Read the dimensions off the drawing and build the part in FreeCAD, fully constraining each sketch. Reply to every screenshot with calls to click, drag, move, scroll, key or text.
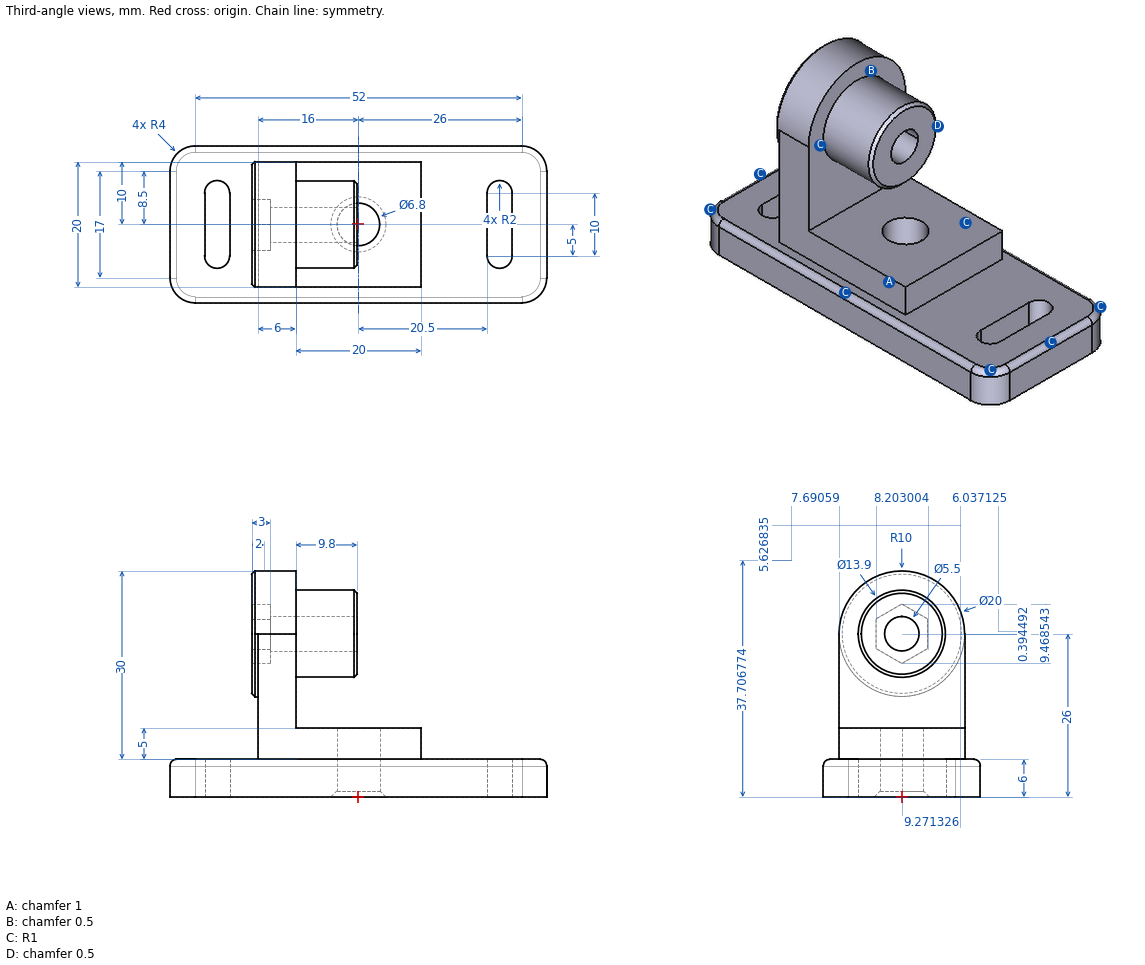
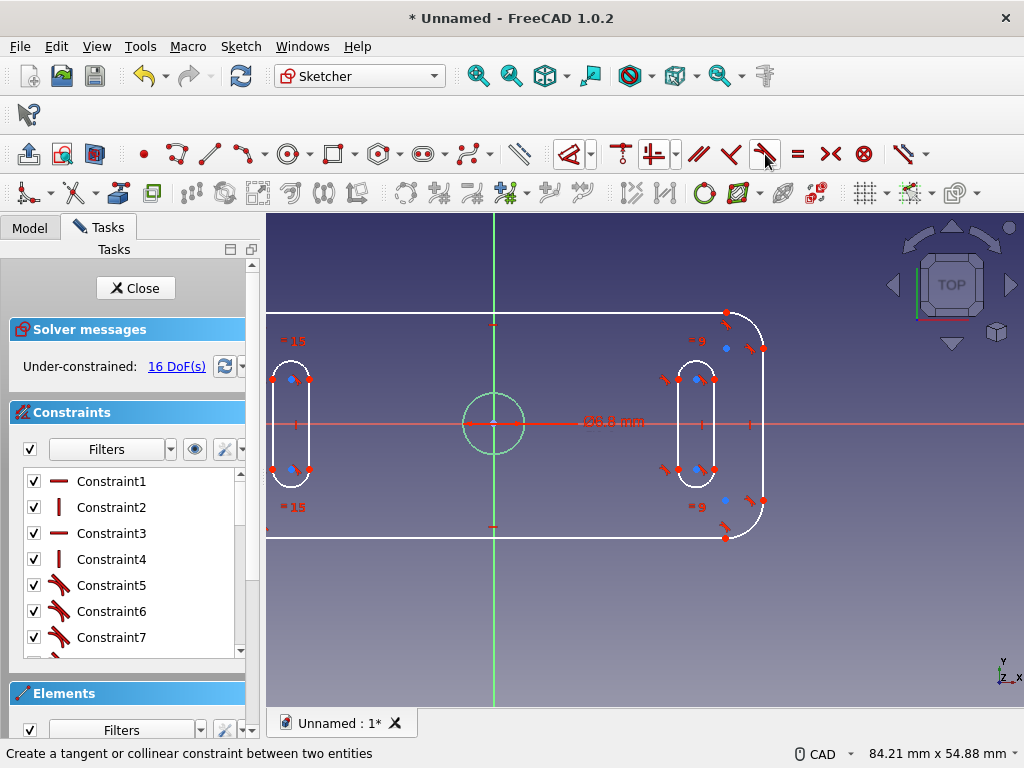
scroll(745, 534, down, 2)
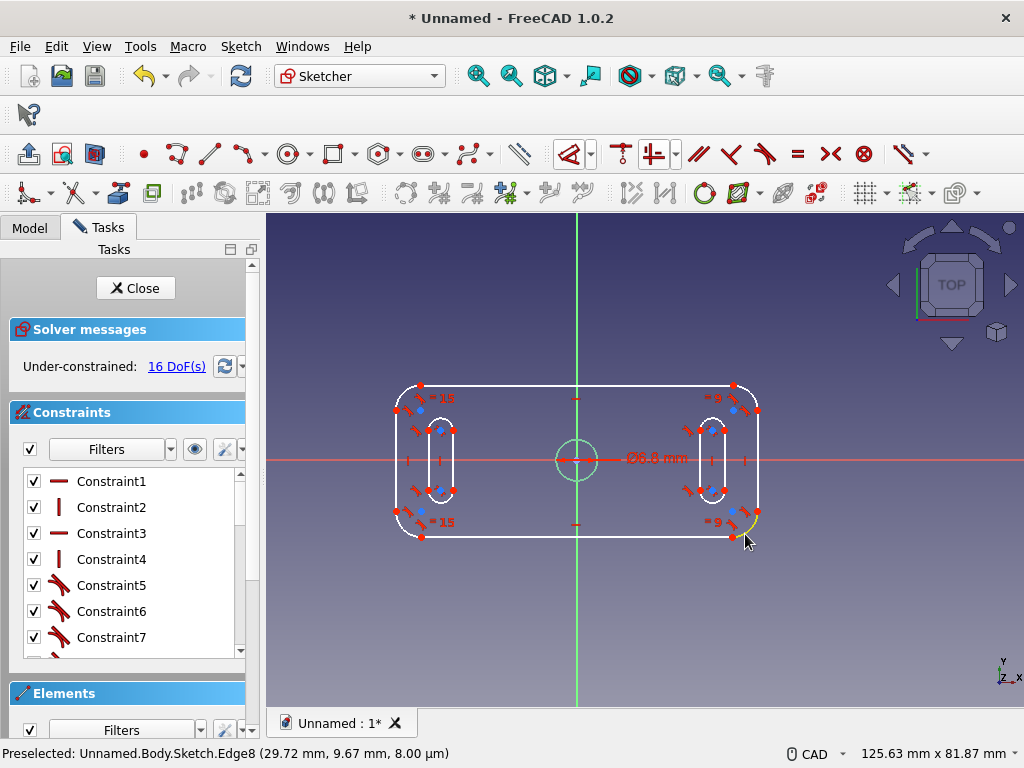
click(409, 388)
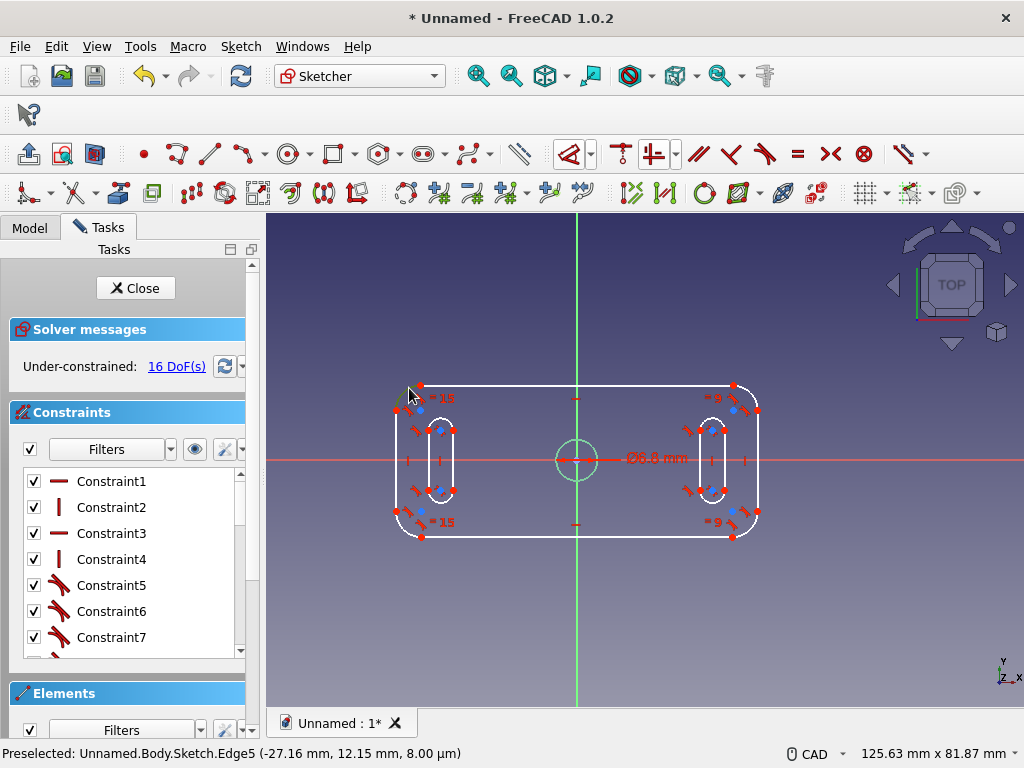
click(399, 523)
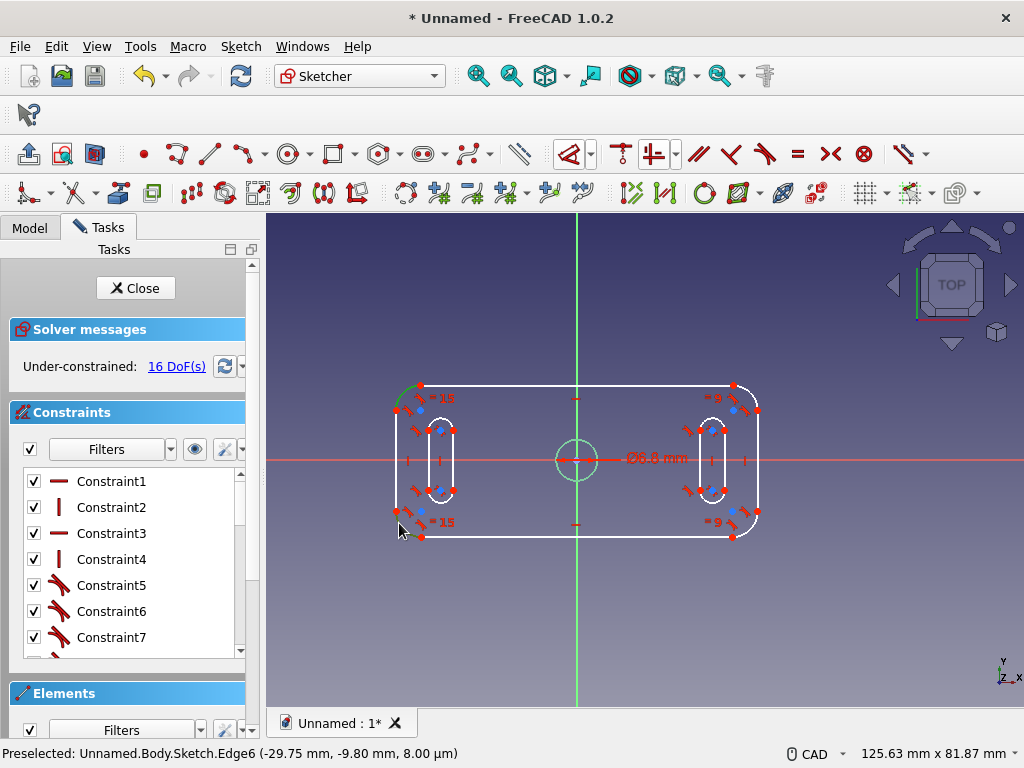
click(744, 534)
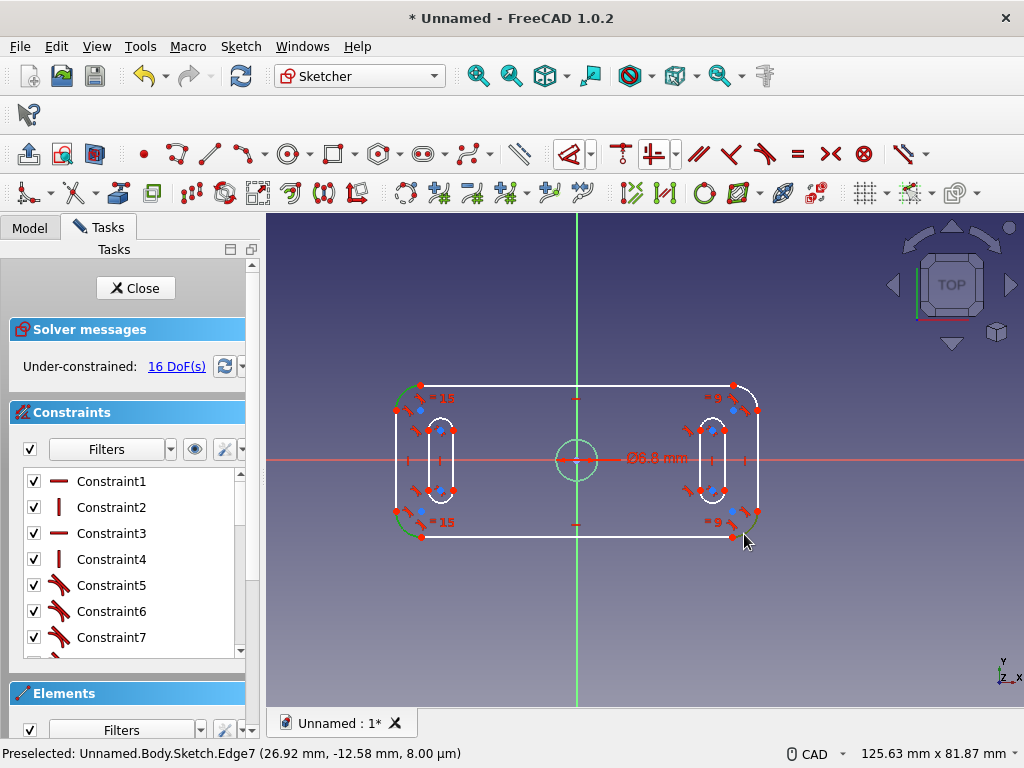
click(755, 399)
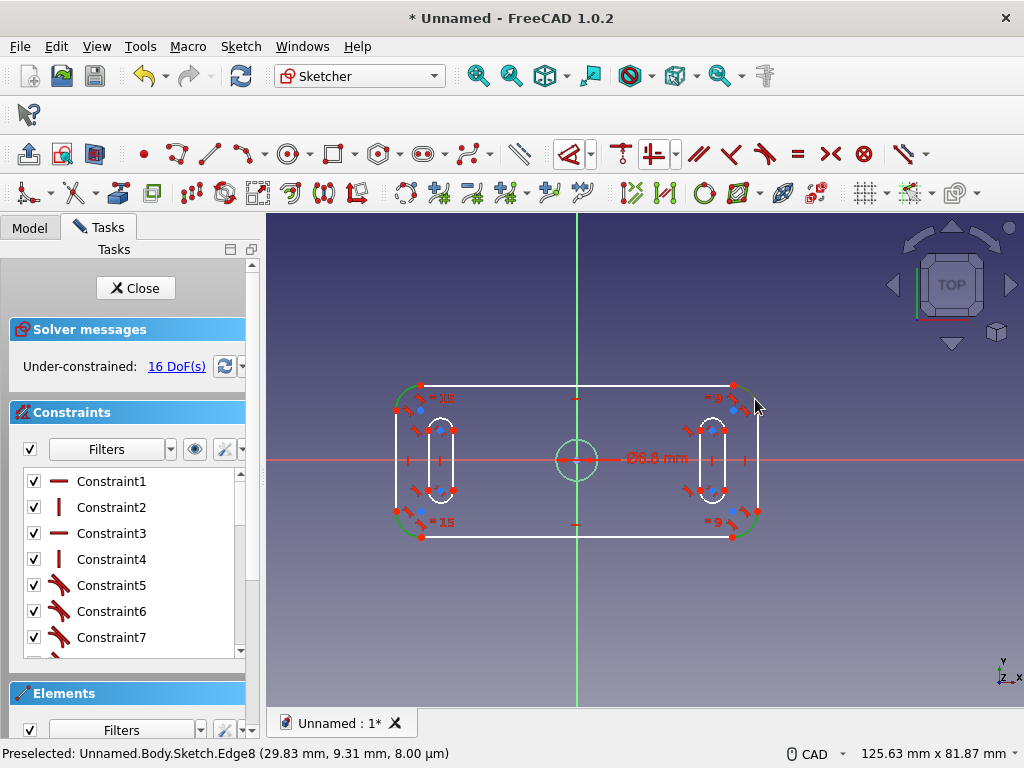
click(798, 154)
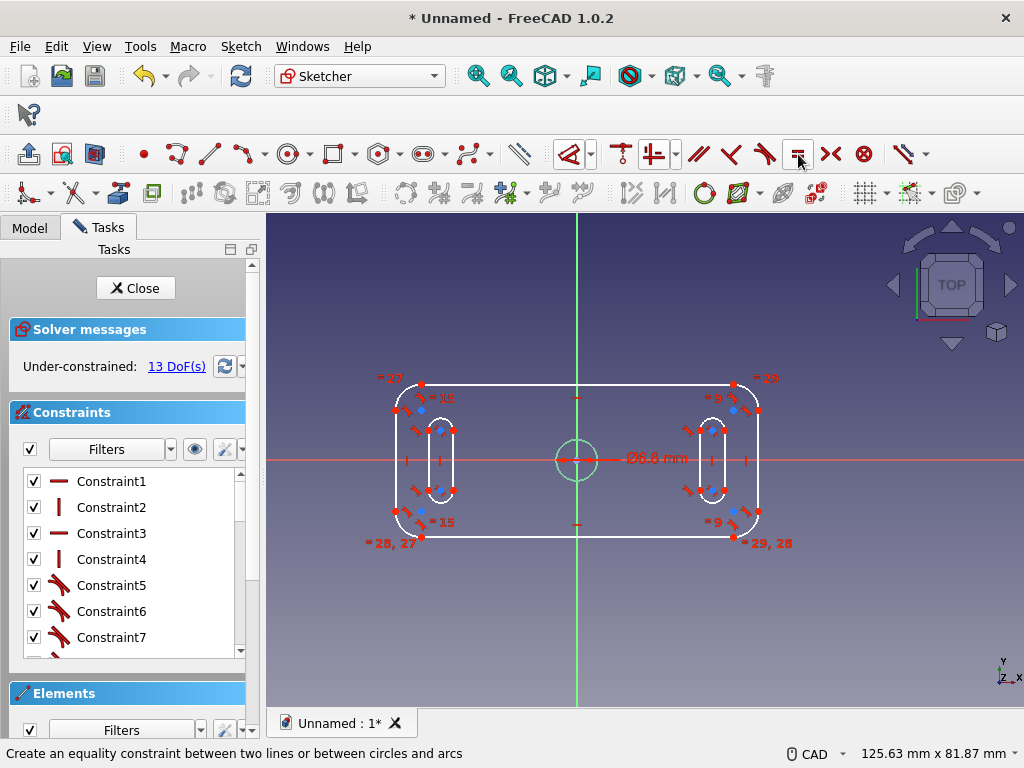
scroll(705, 501, up, 2)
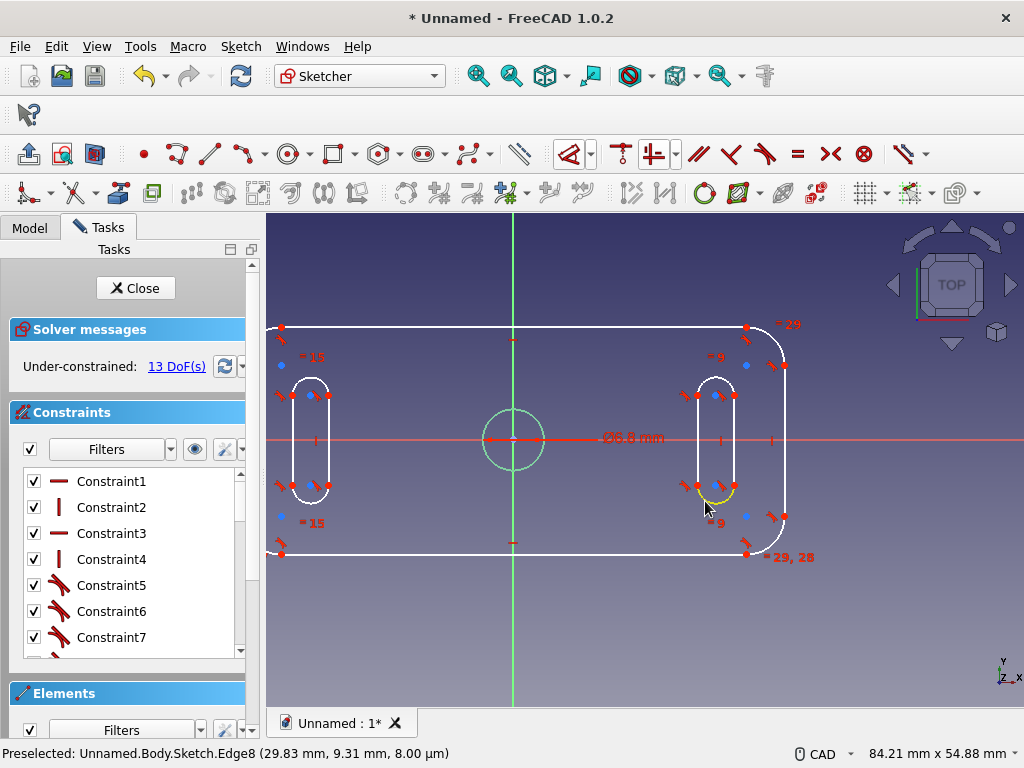
click(705, 500)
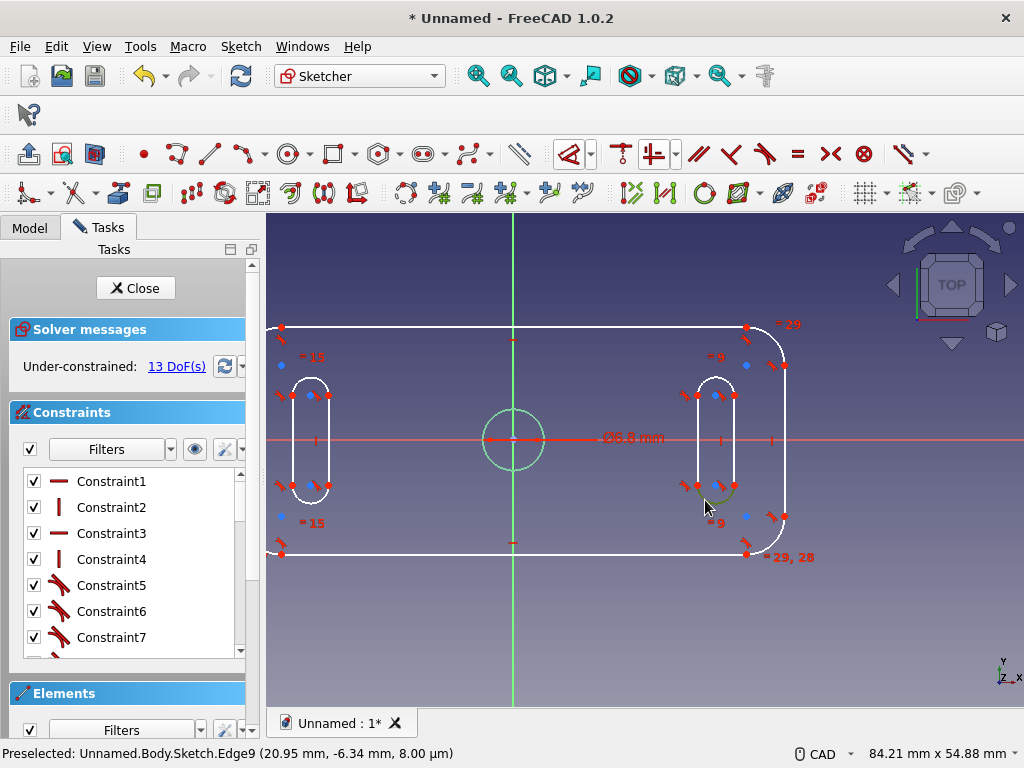
click(300, 500)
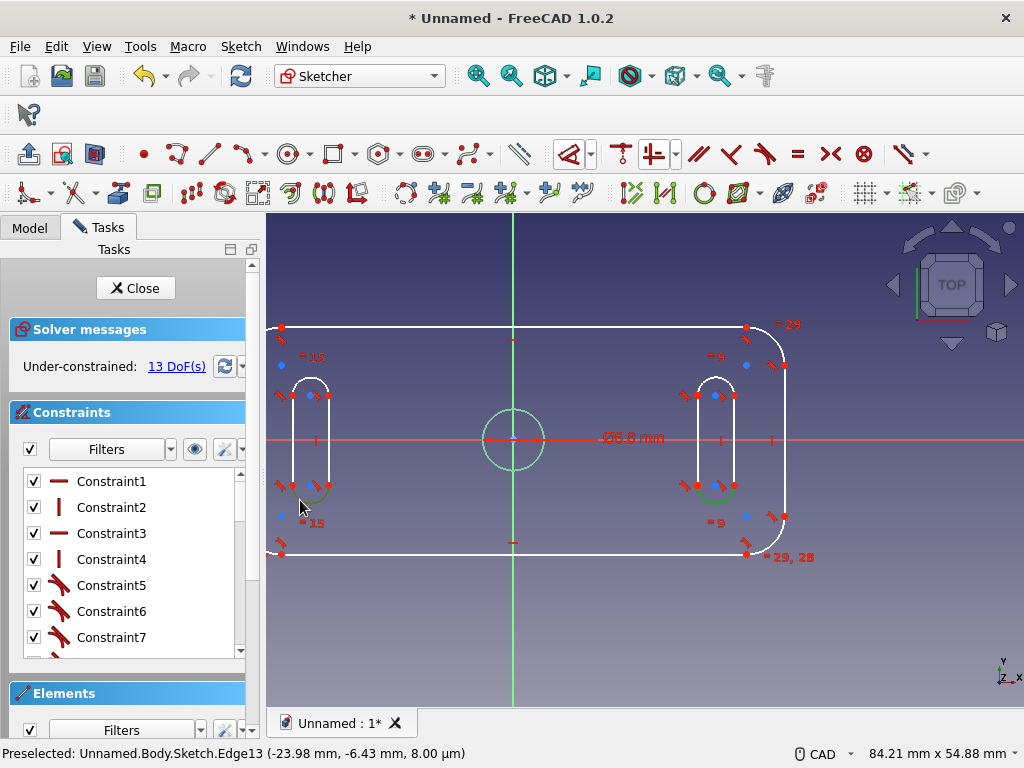
click(798, 154)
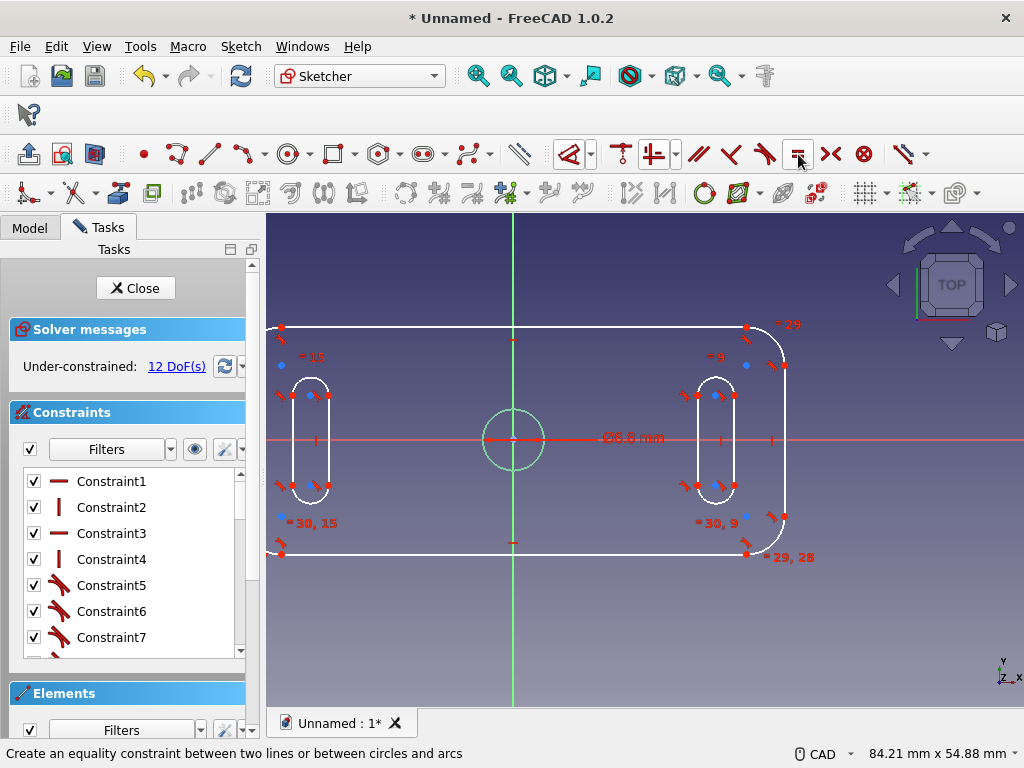
click(716, 486)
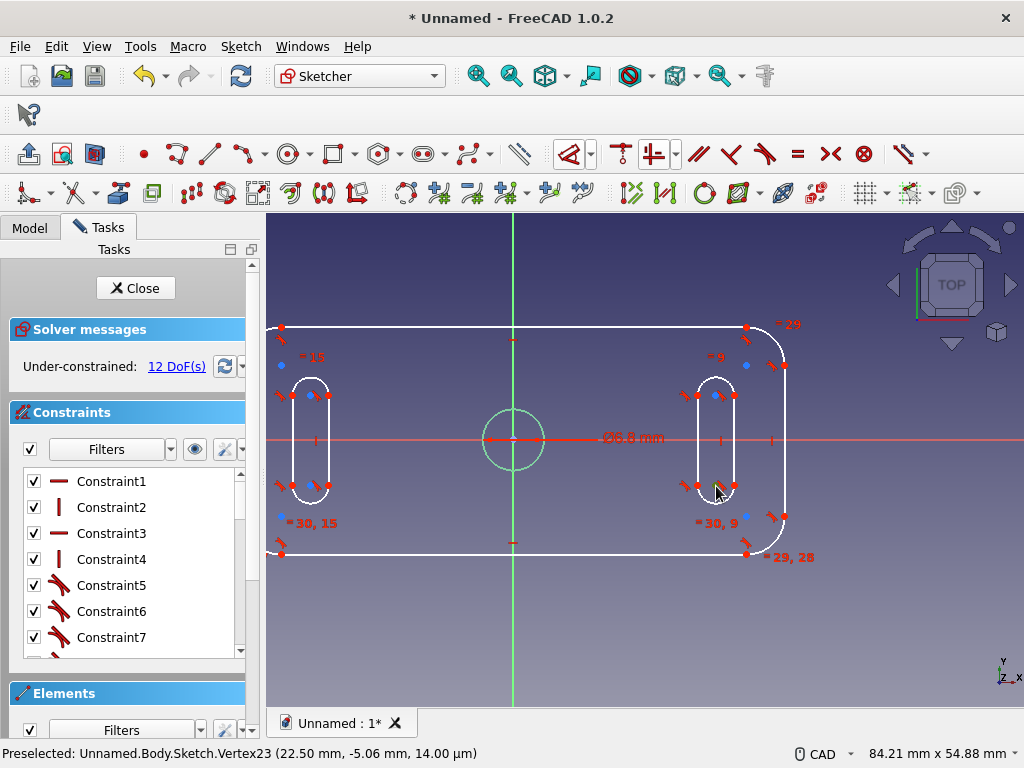
click(311, 485)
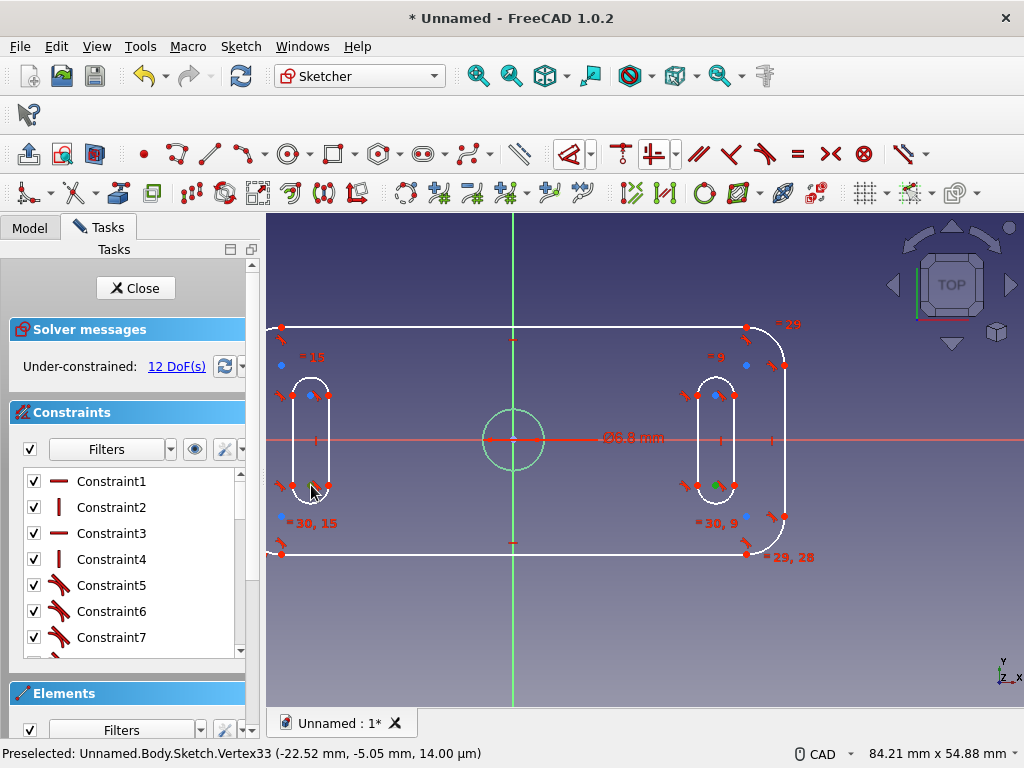
click(513, 648)